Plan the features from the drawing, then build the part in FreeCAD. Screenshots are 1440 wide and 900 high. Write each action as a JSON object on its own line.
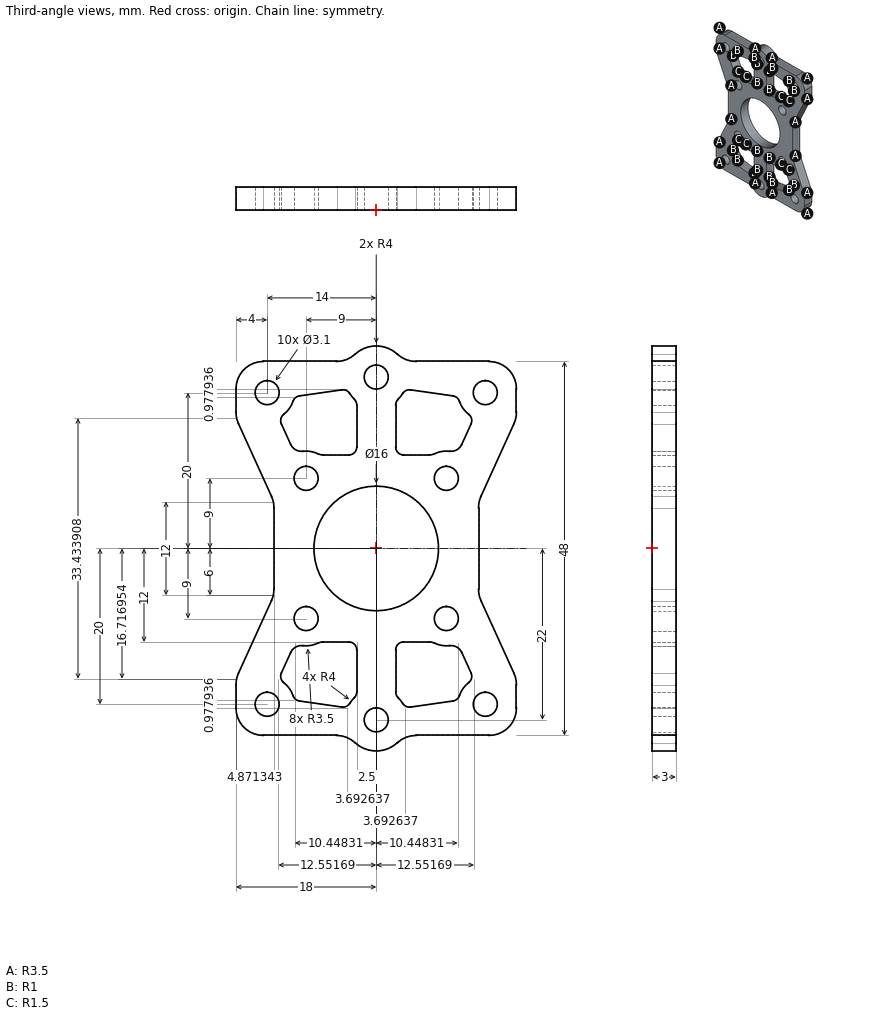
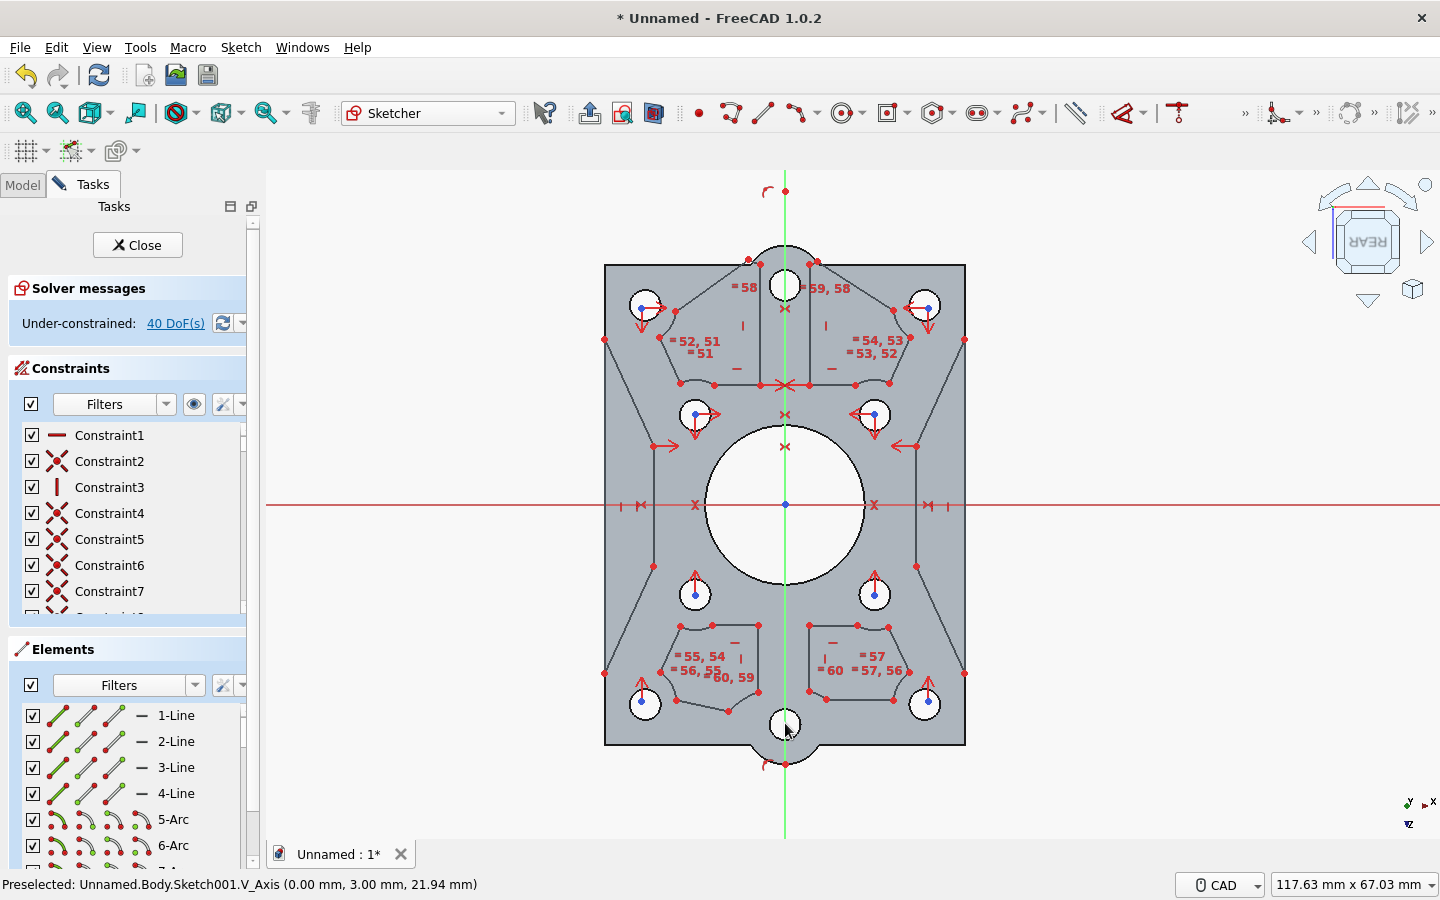
{"action": "left_click", "coordinate": [605, 673]}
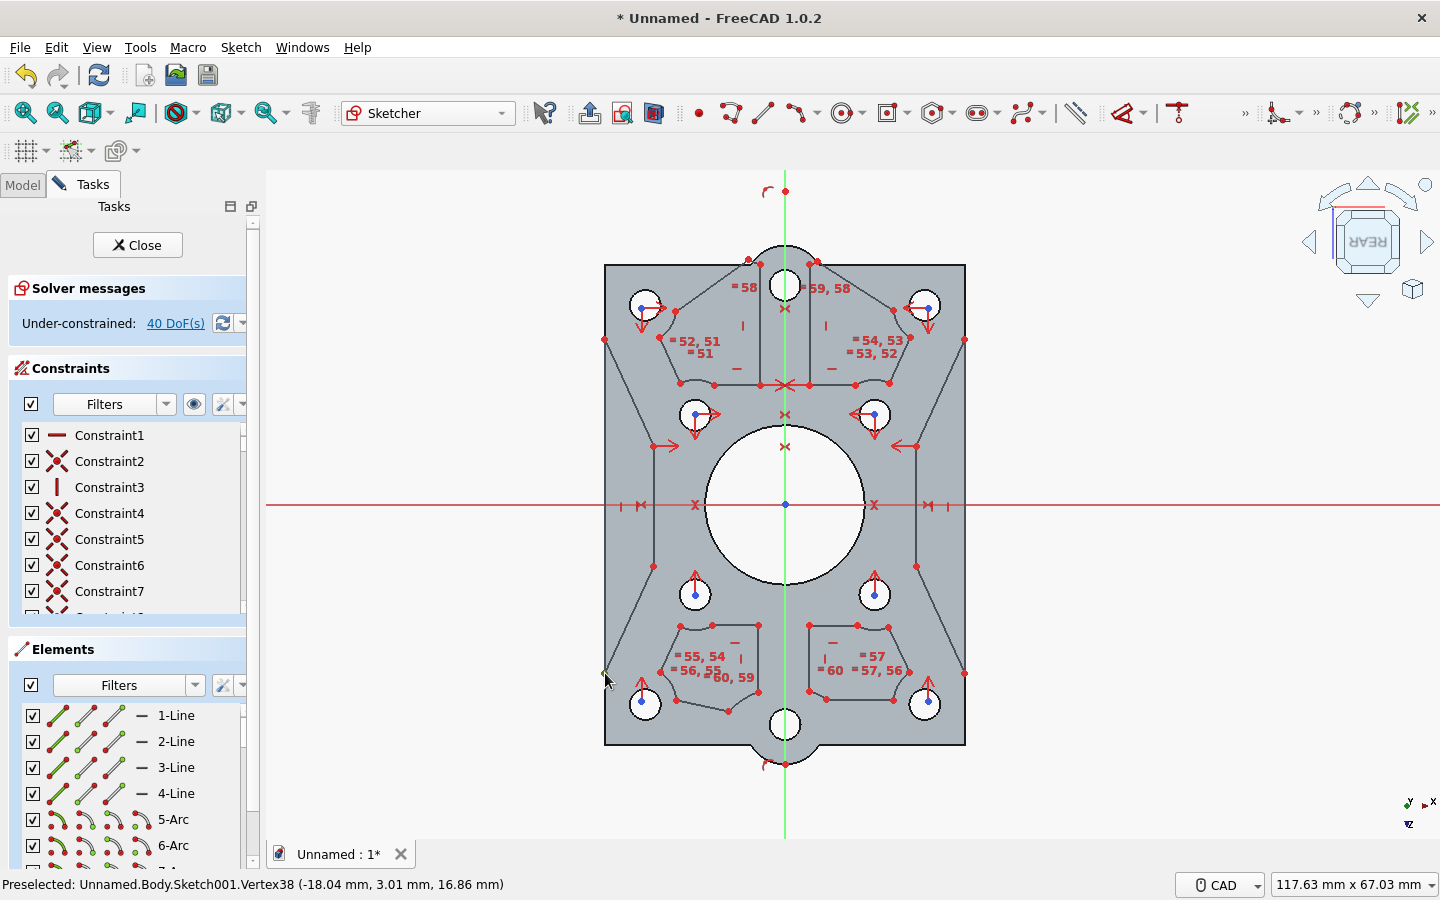
{"action": "left_click", "coordinate": [965, 673]}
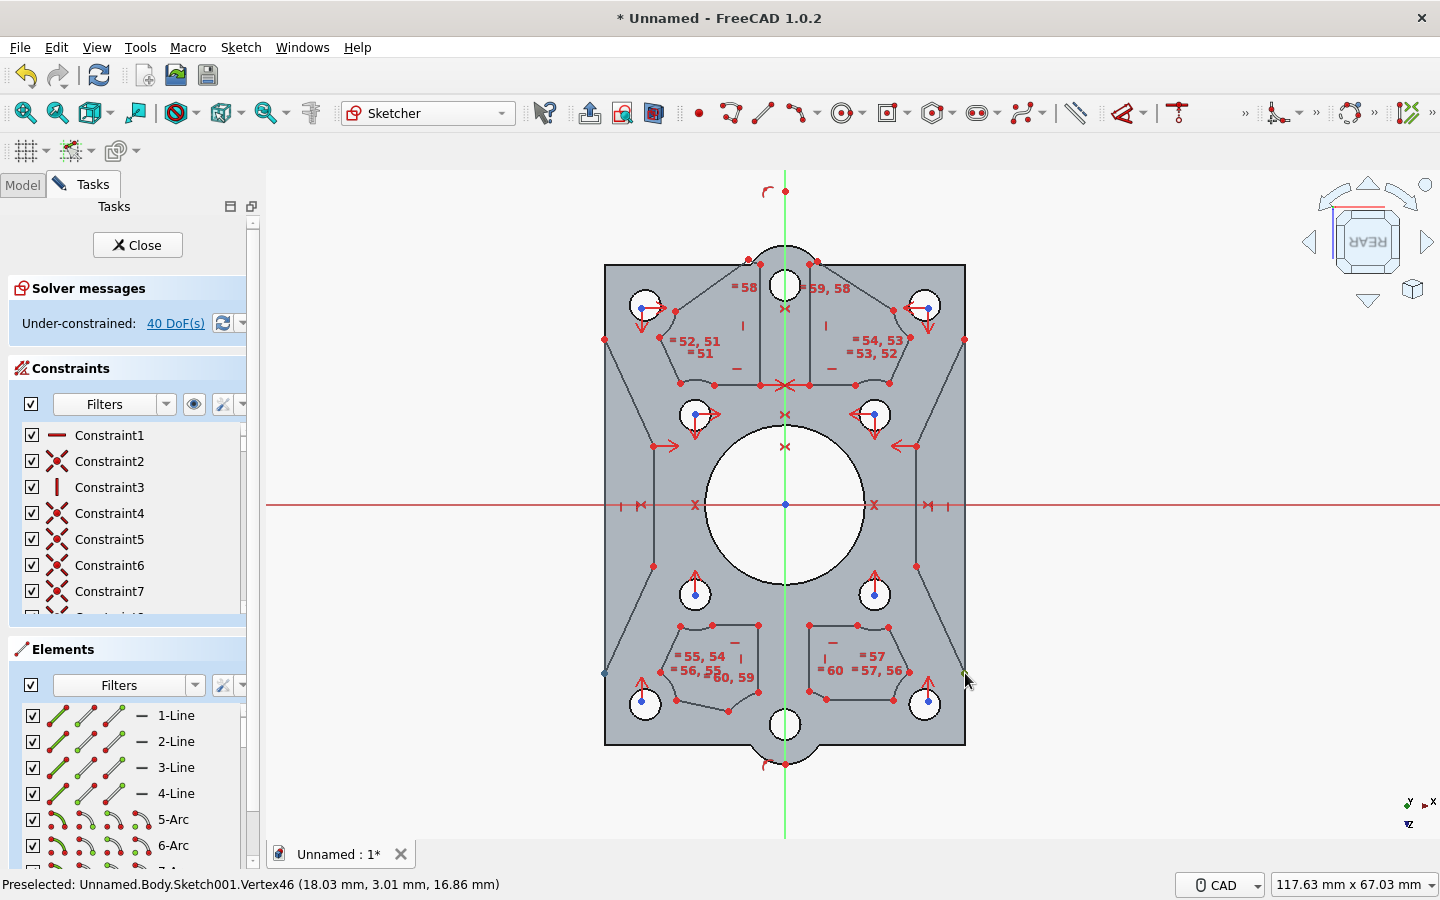
{"action": "left_click", "coordinate": [785, 723]}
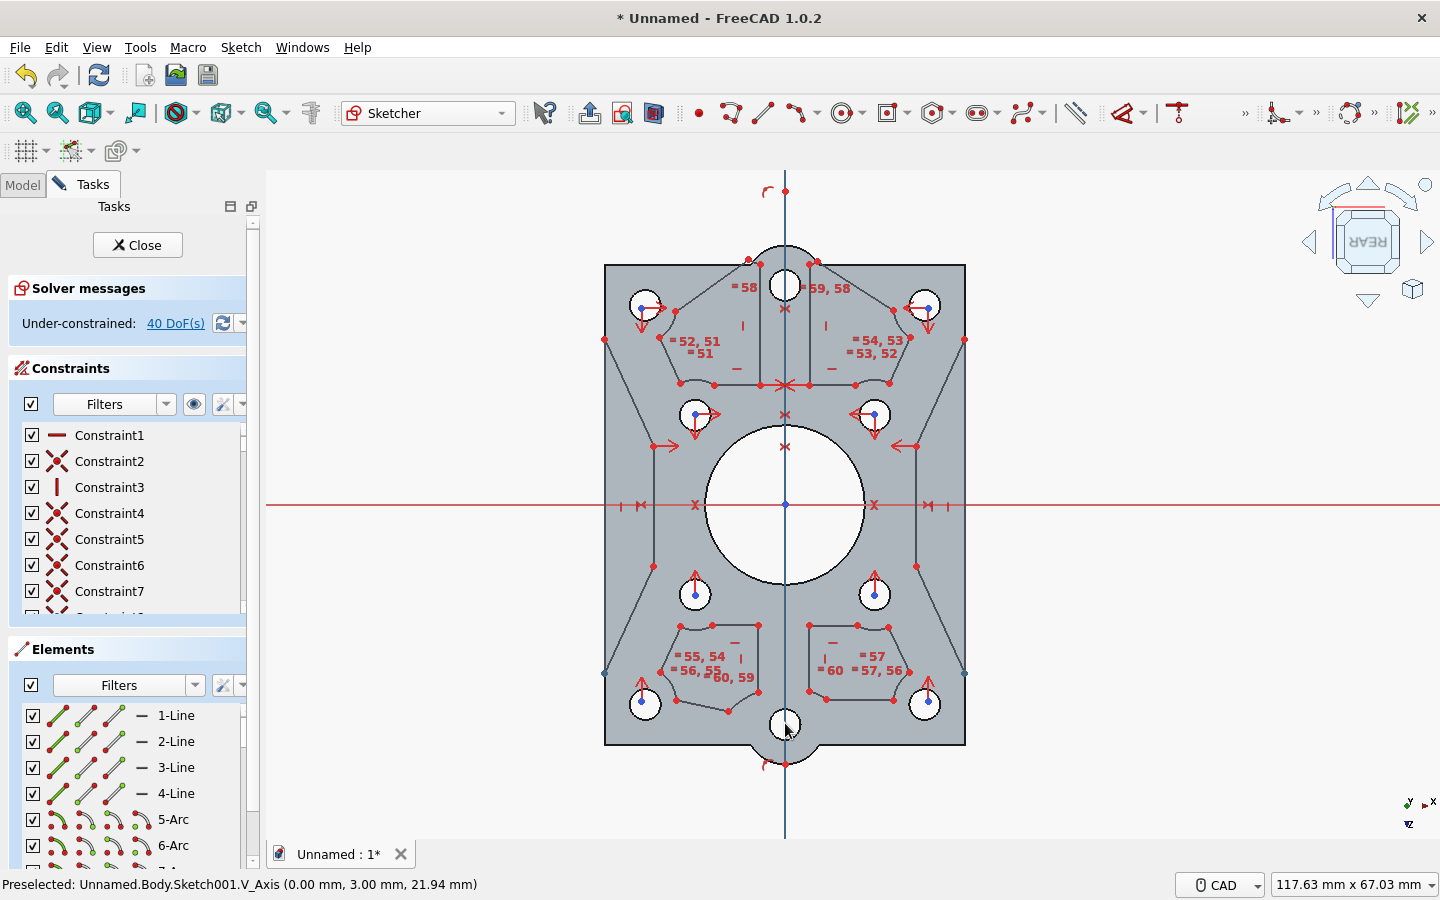
{"action": "key", "text": "s"}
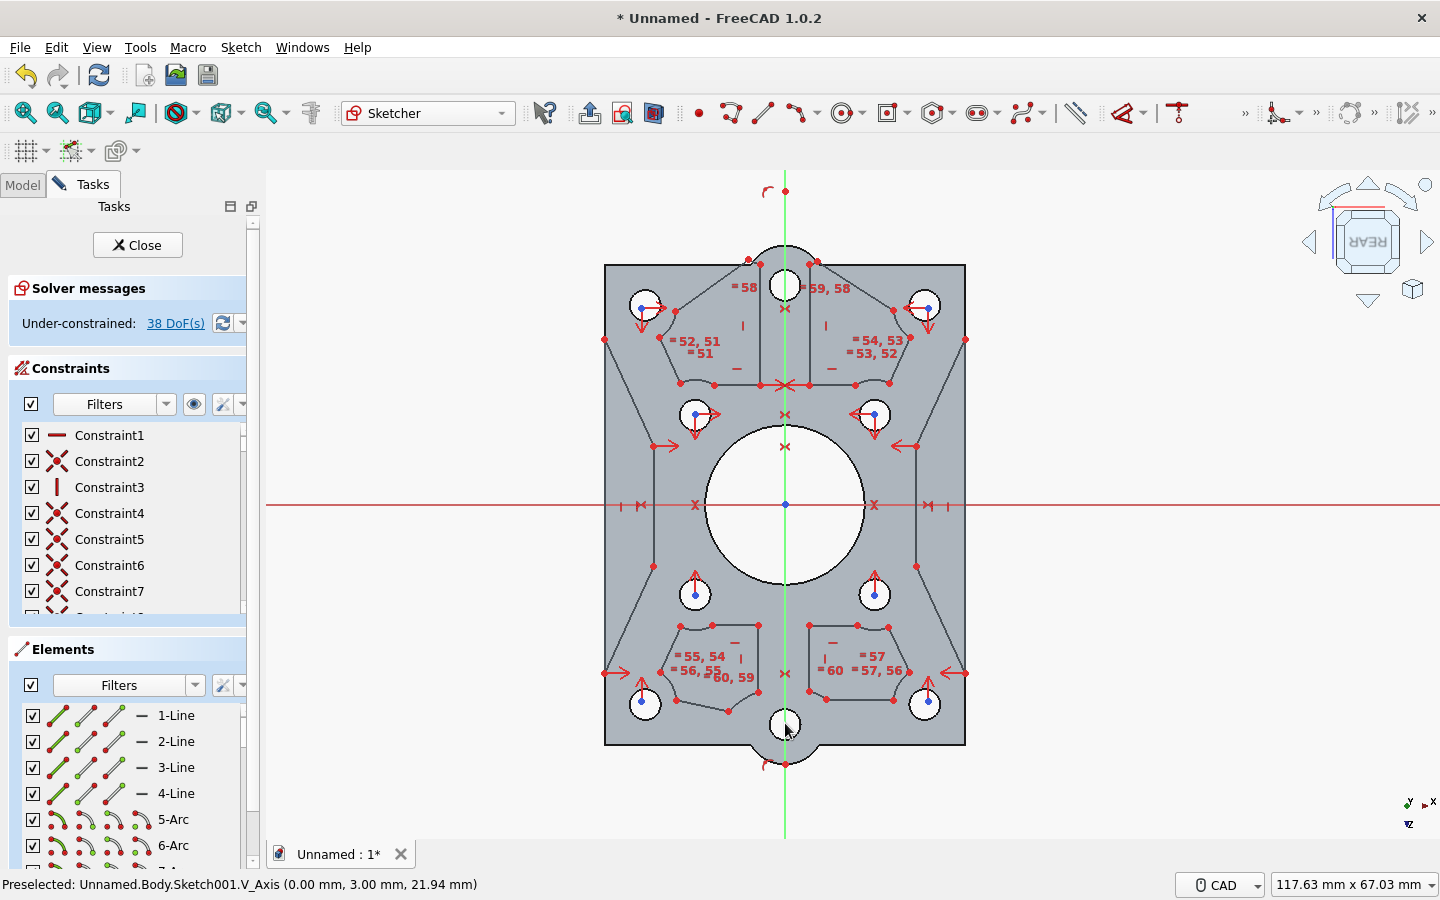
{"action": "left_click", "coordinate": [749, 260]}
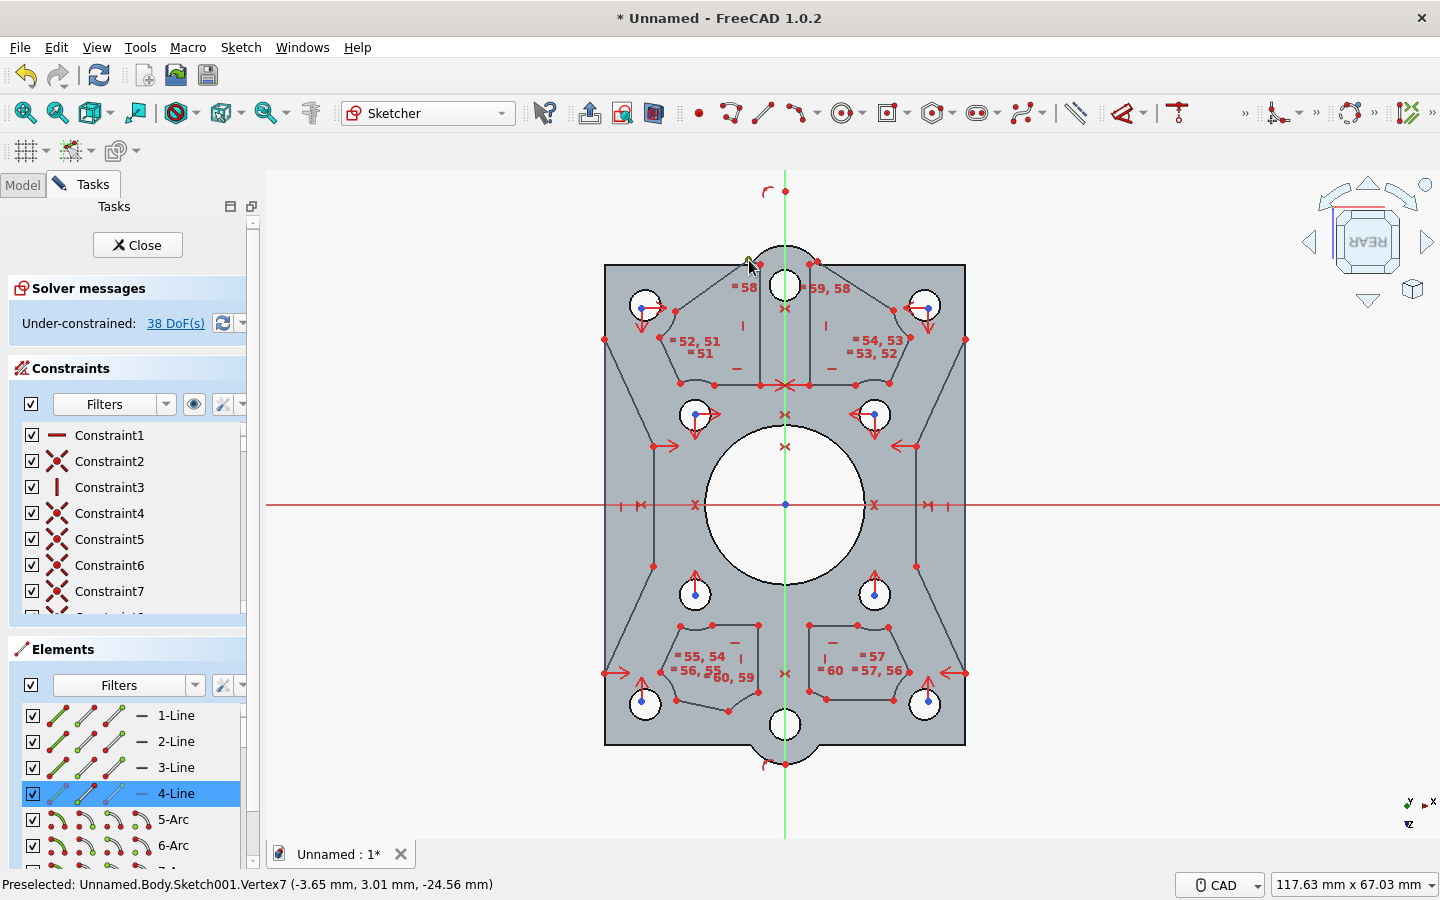
{"action": "left_click", "coordinate": [729, 712]}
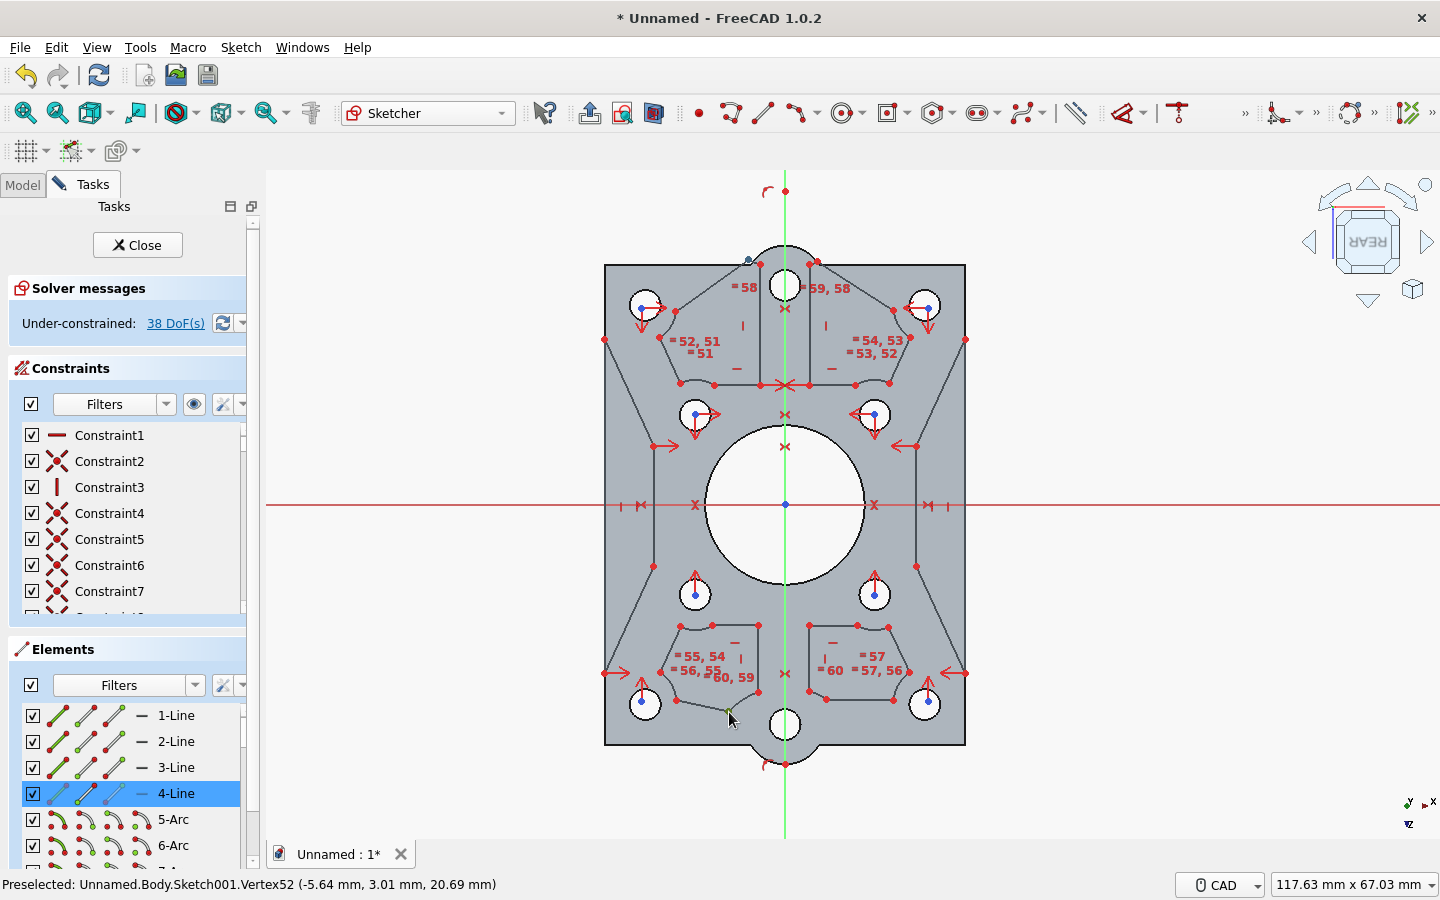
{"action": "left_click", "coordinate": [364, 505]}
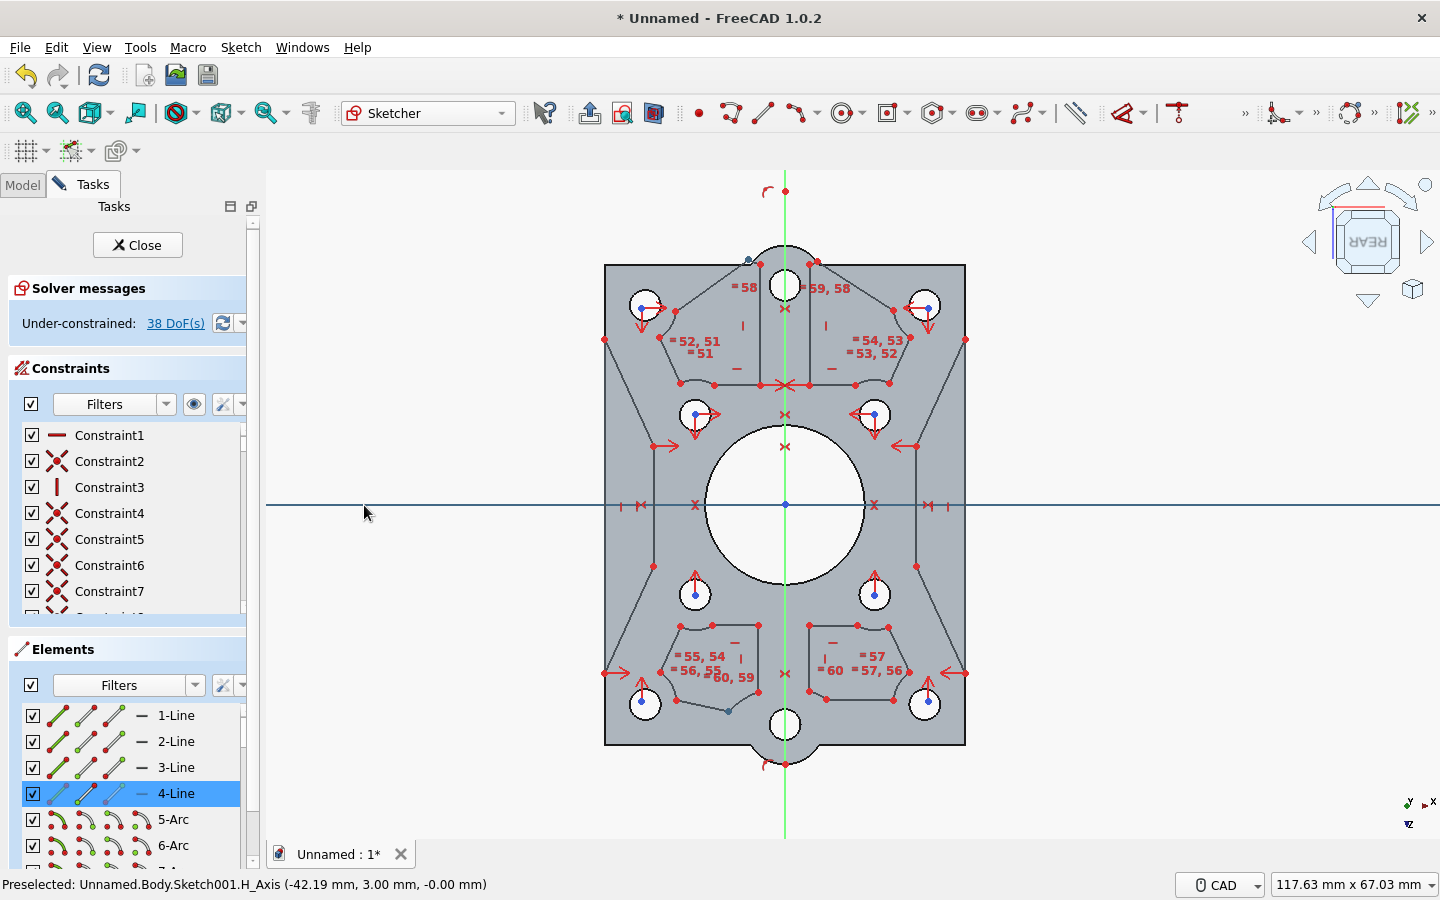
{"action": "key", "text": "s"}